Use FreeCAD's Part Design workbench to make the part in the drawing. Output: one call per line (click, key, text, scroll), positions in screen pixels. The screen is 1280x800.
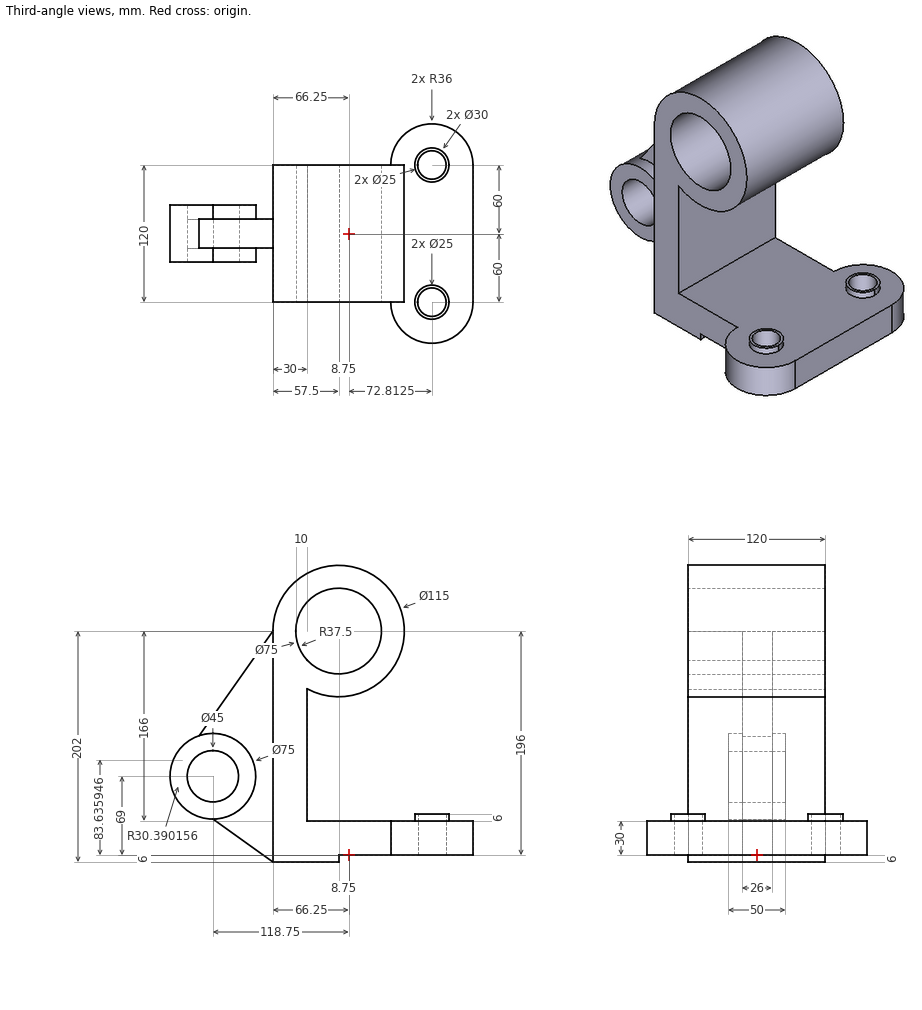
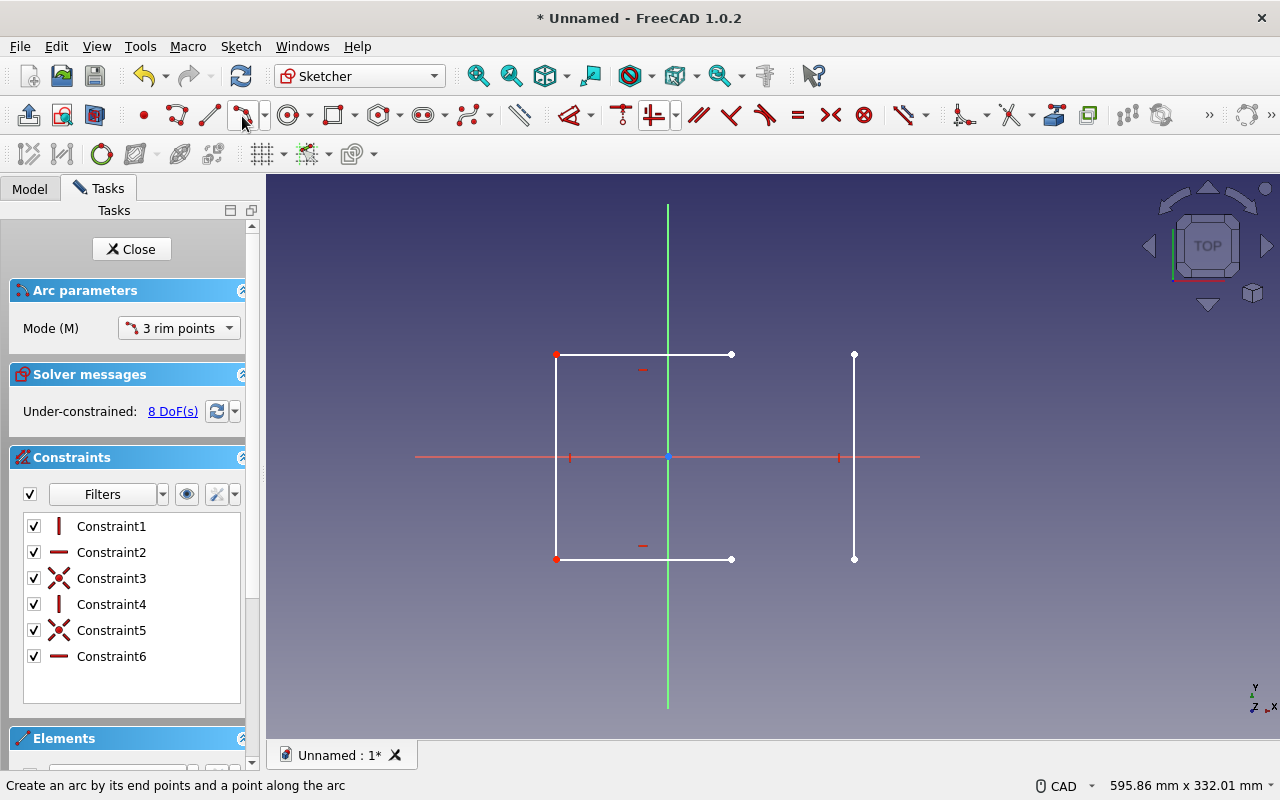
click(854, 355)
click(731, 355)
click(792, 293)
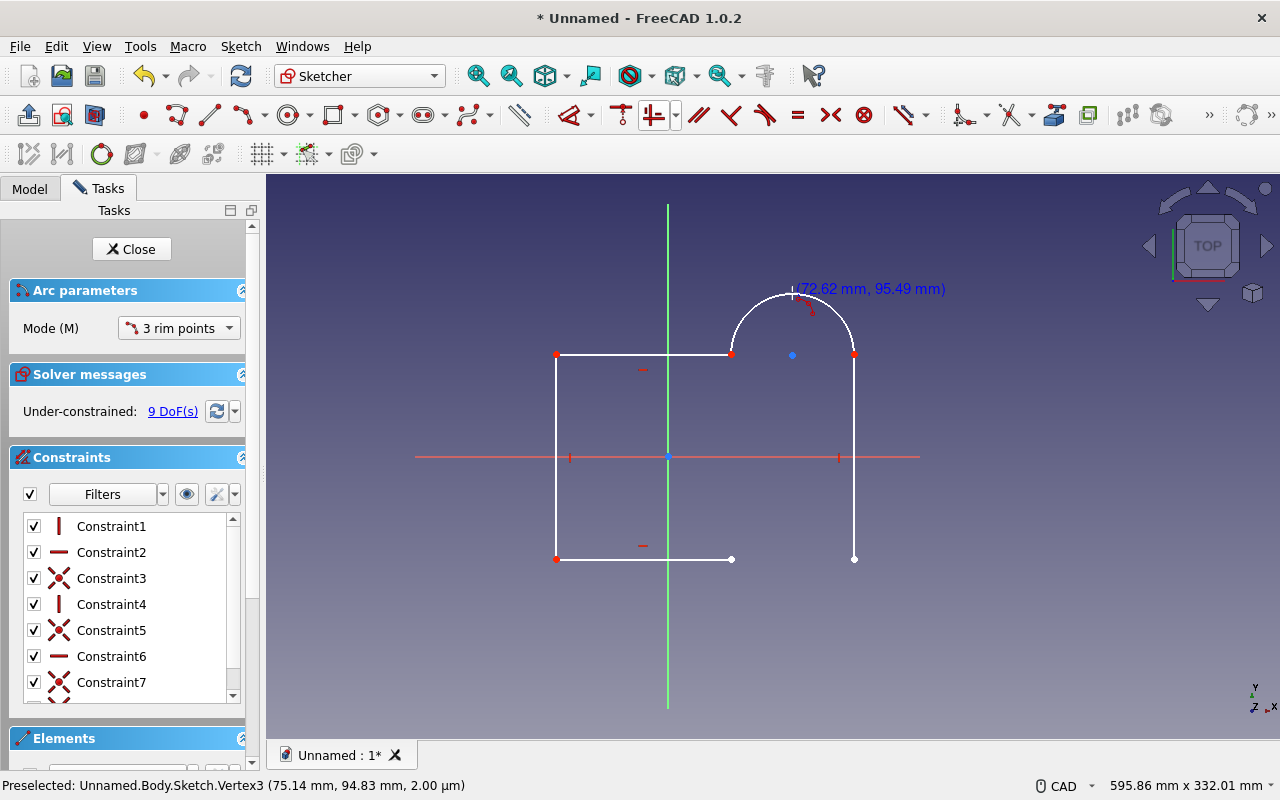
click(731, 560)
click(854, 560)
click(792, 620)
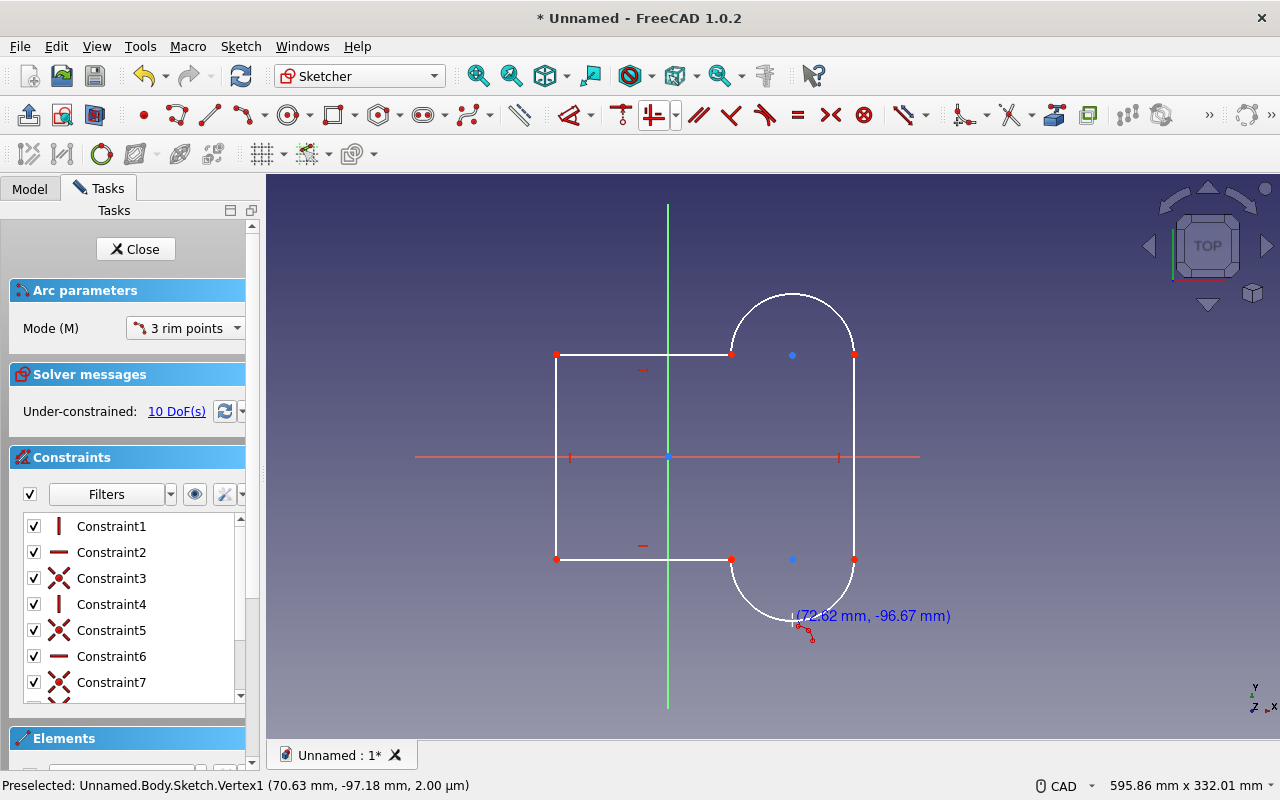
click(288, 116)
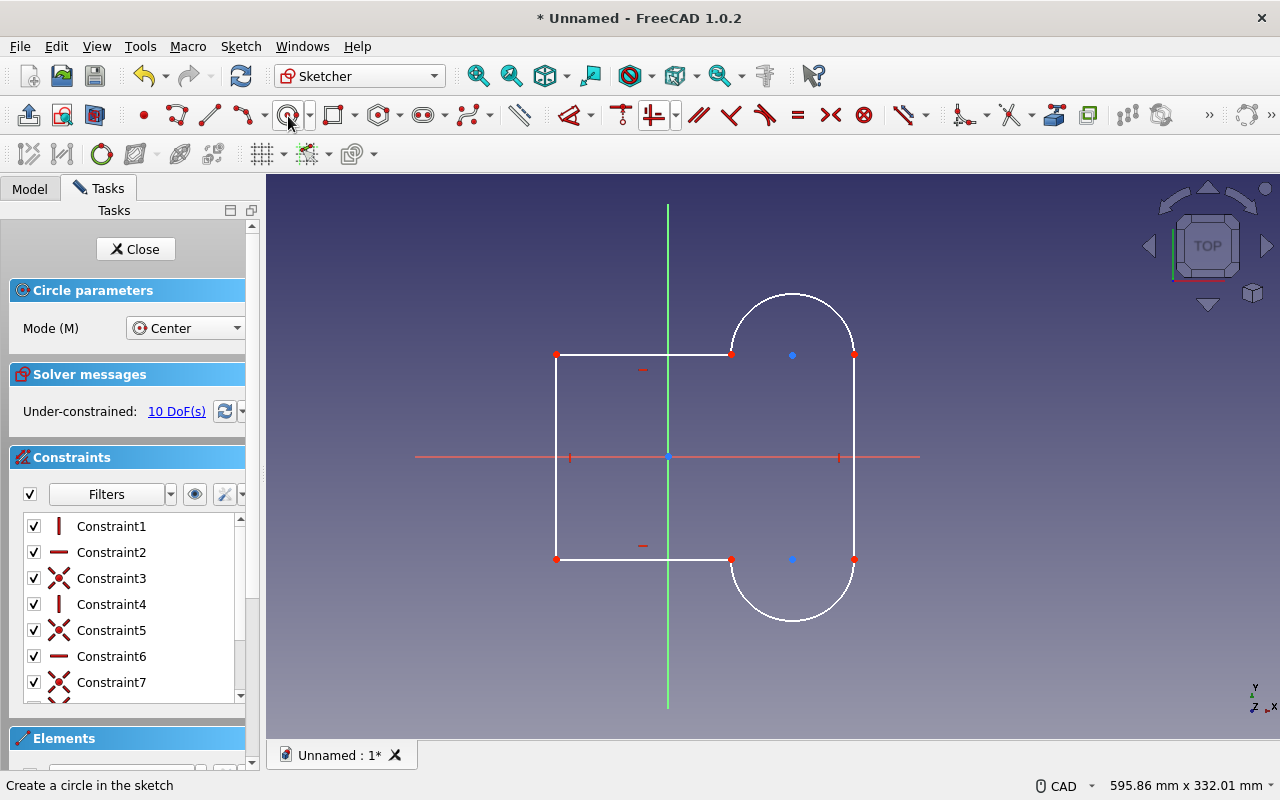
click(792, 559)
click(807, 544)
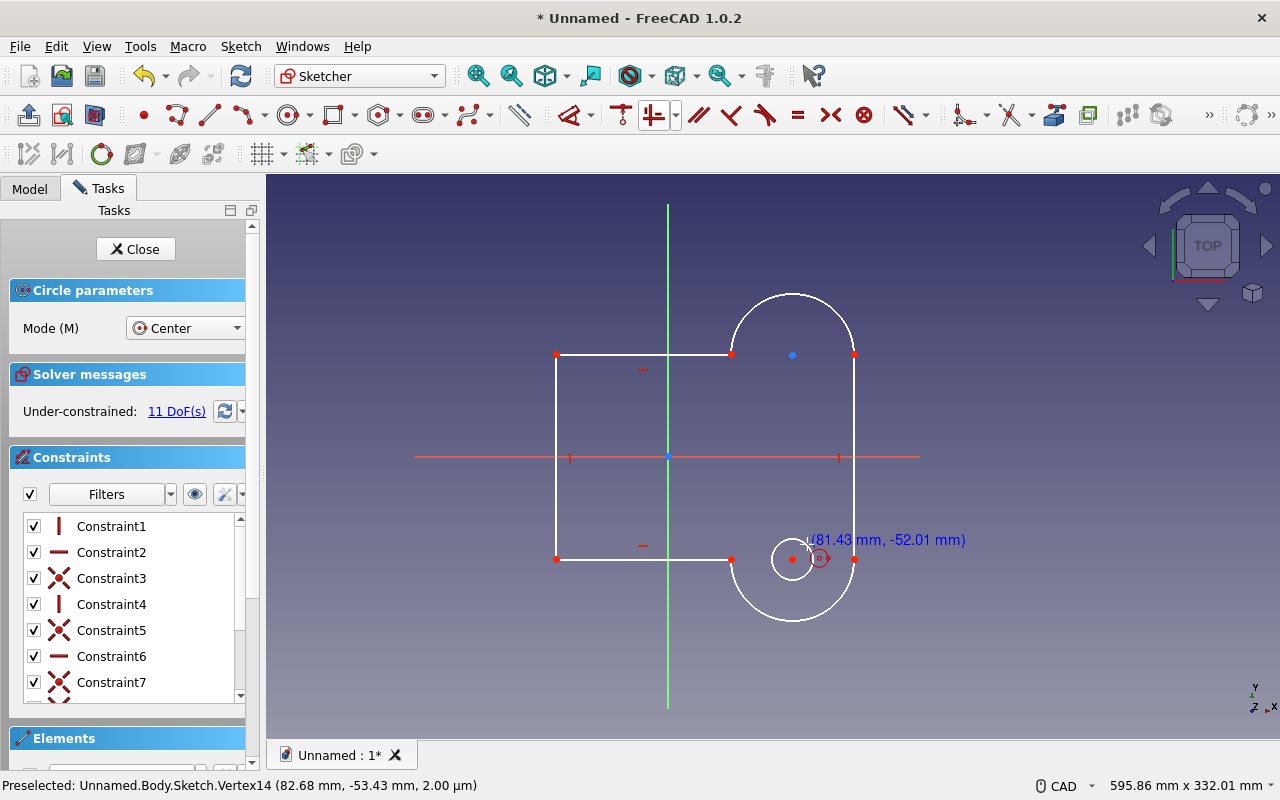
click(792, 354)
click(807, 339)
key(Escape)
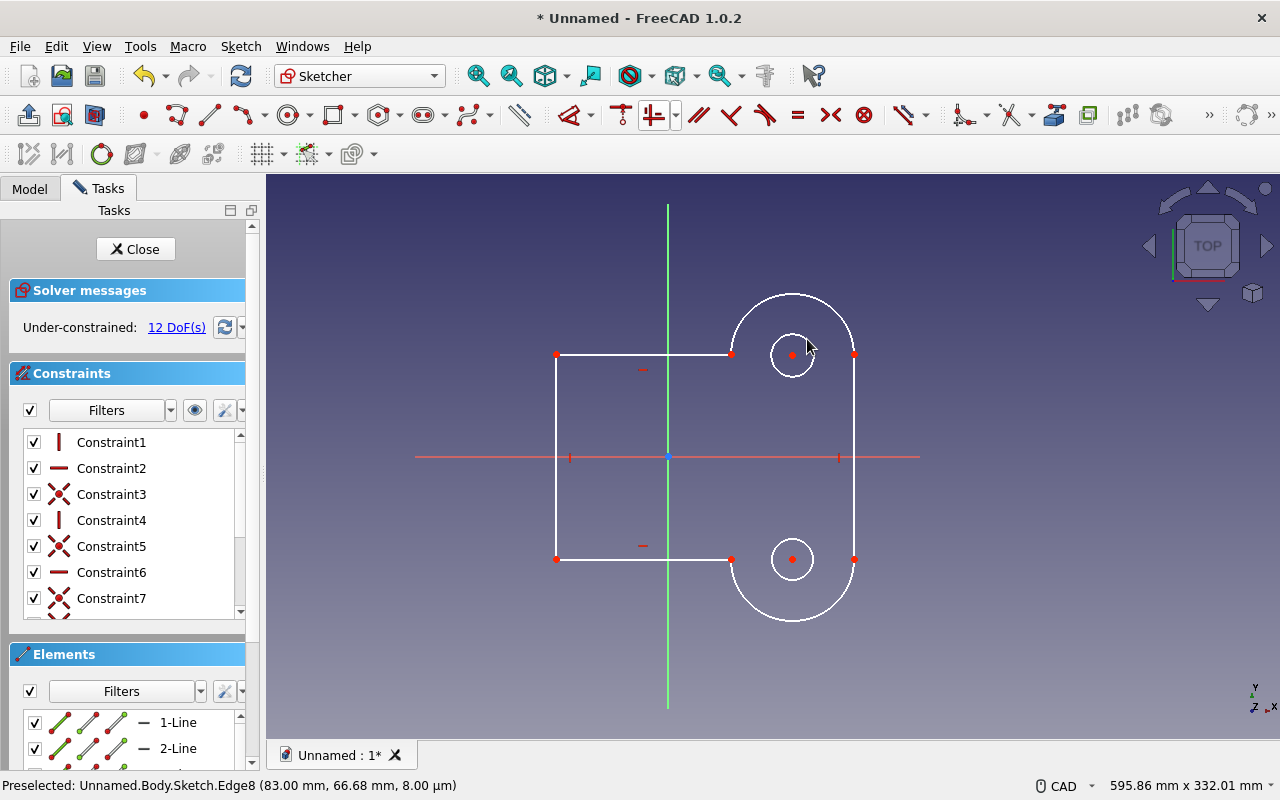
click(854, 499)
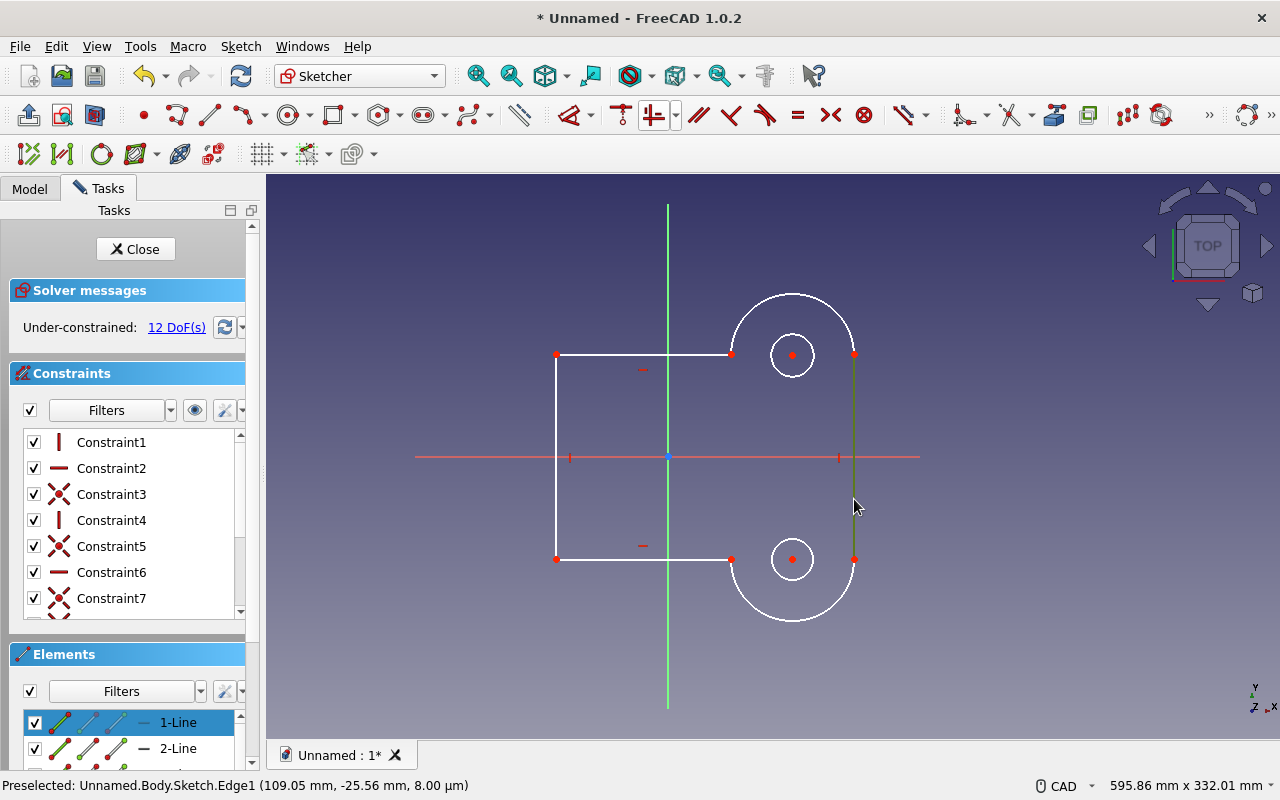
click(828, 306)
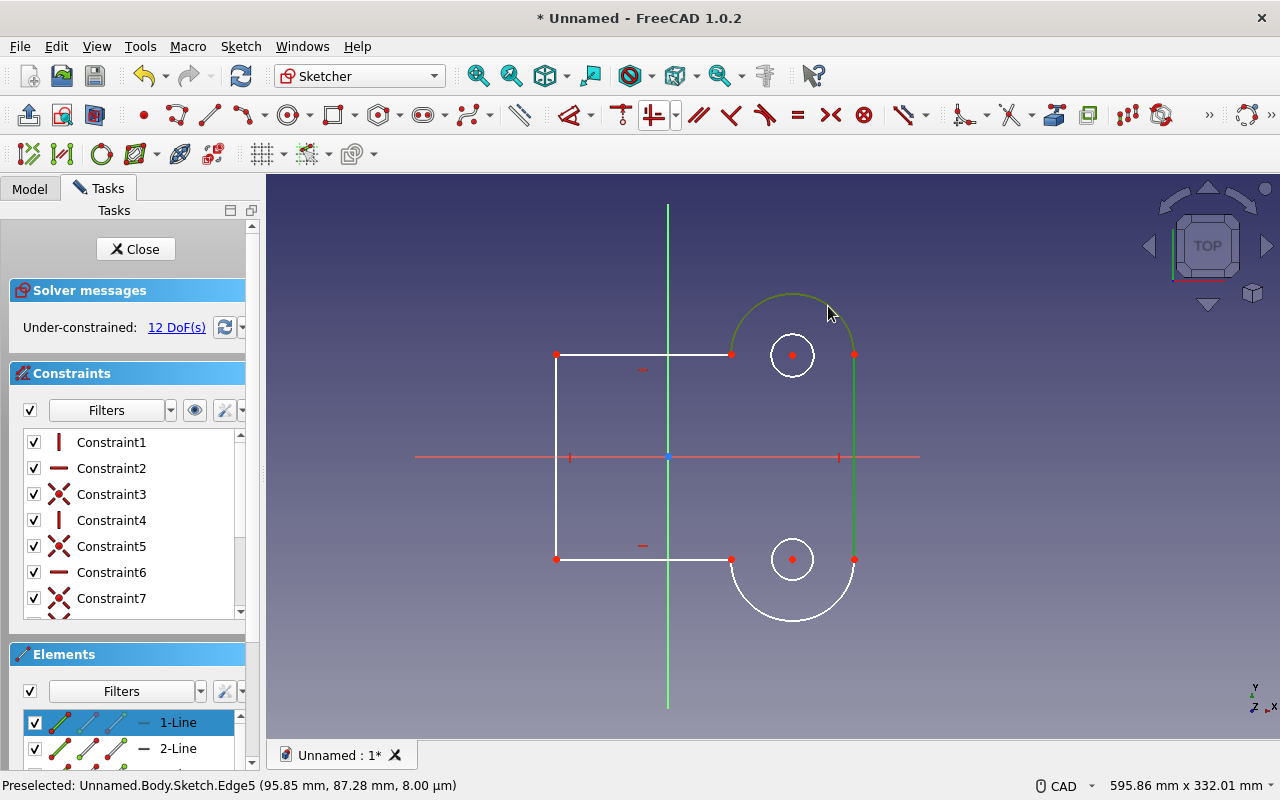
click(765, 116)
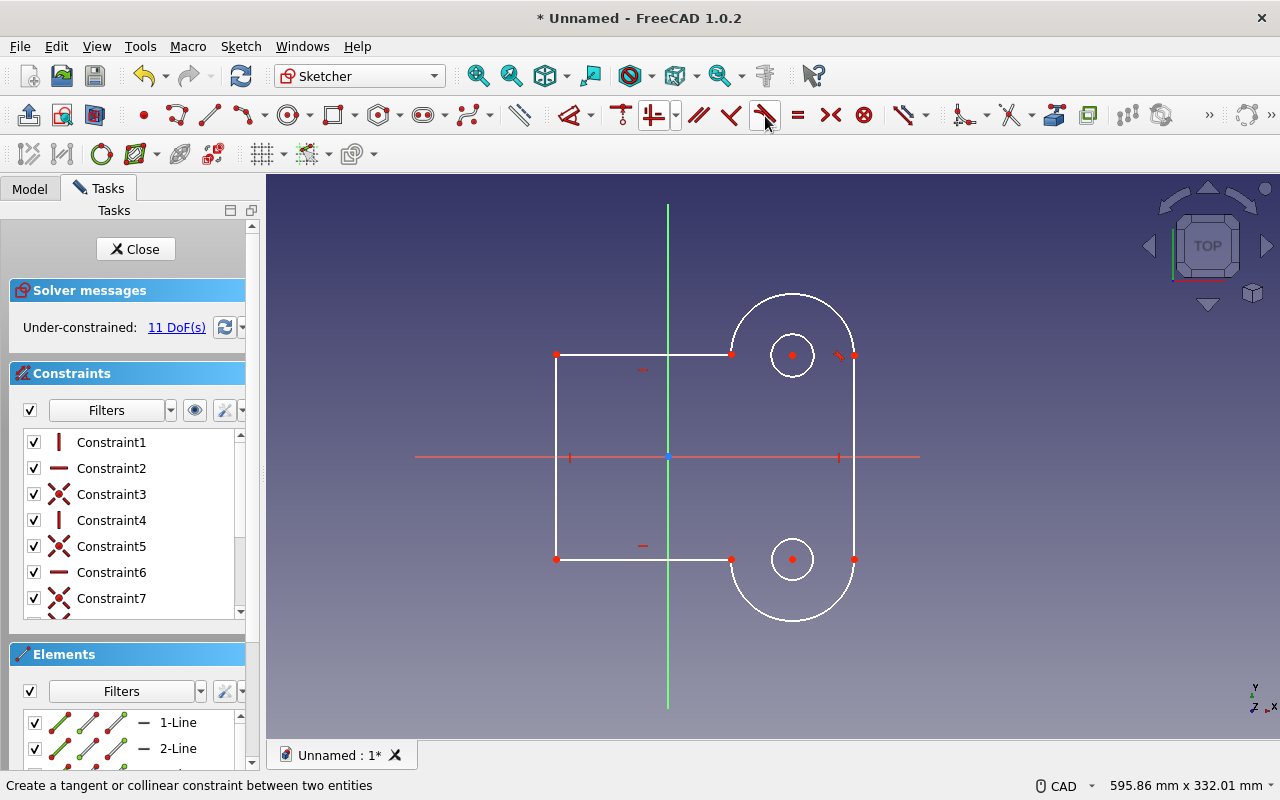
click(854, 499)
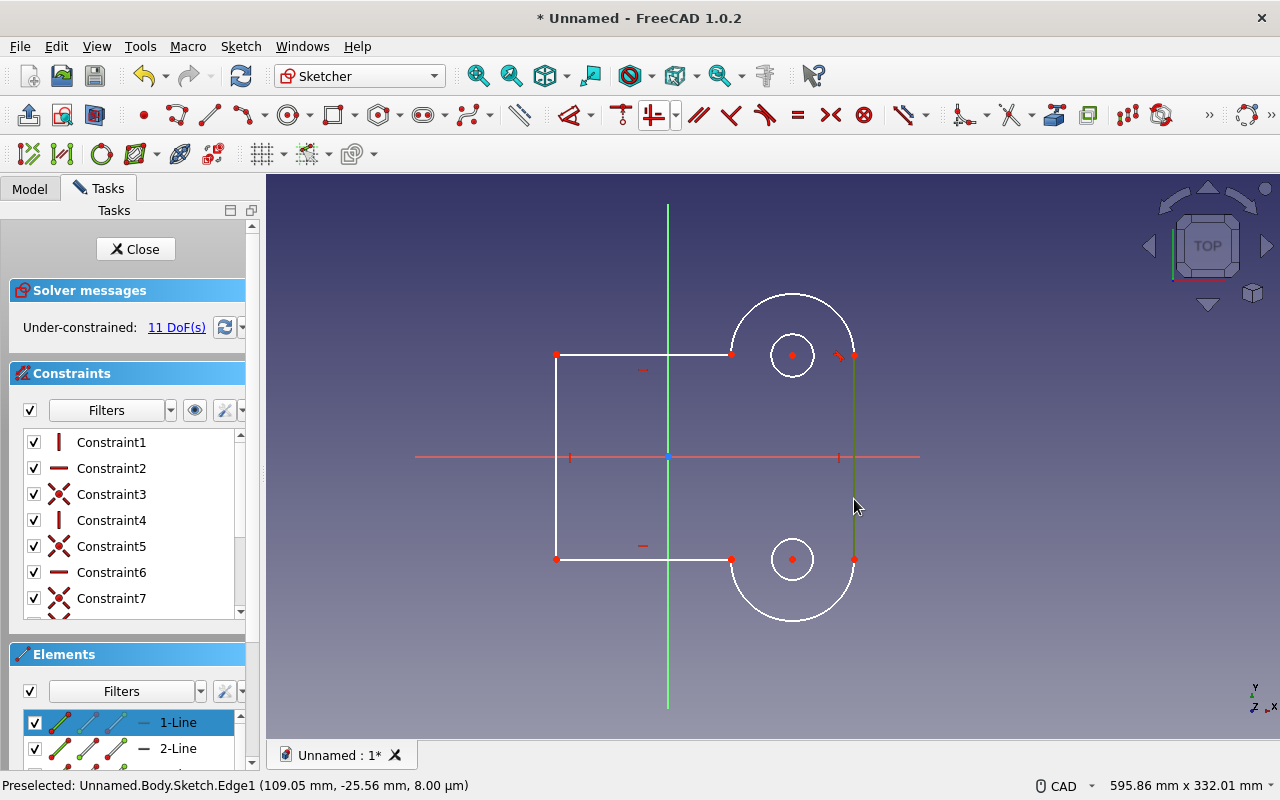
click(757, 609)